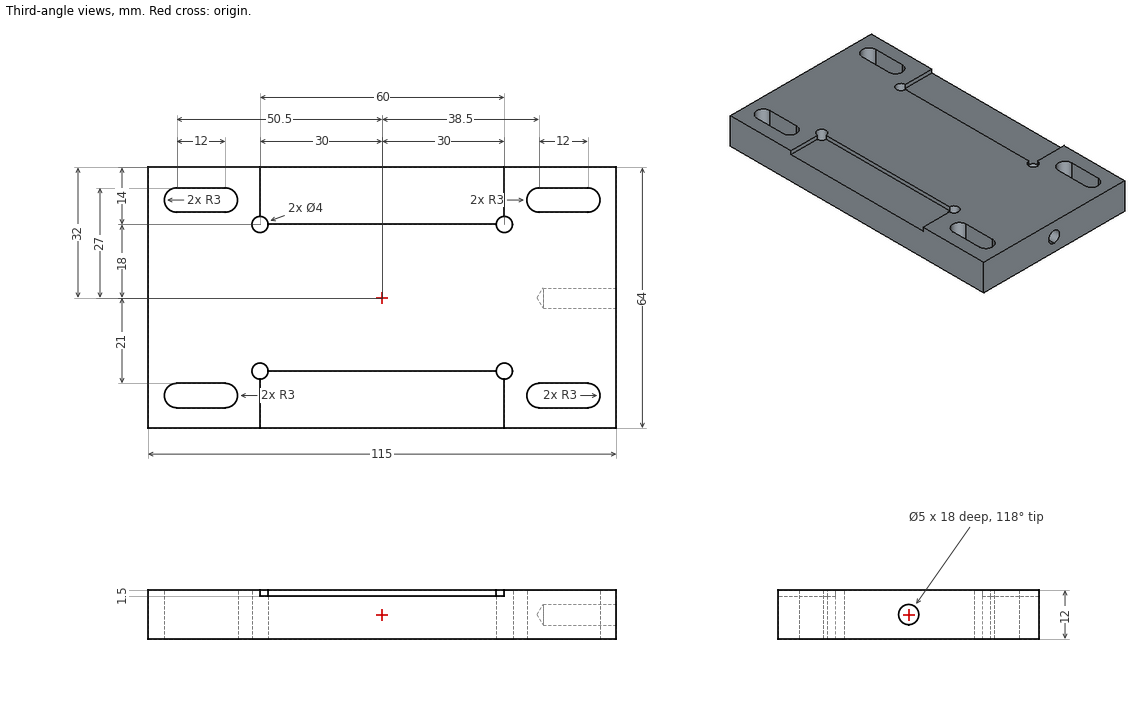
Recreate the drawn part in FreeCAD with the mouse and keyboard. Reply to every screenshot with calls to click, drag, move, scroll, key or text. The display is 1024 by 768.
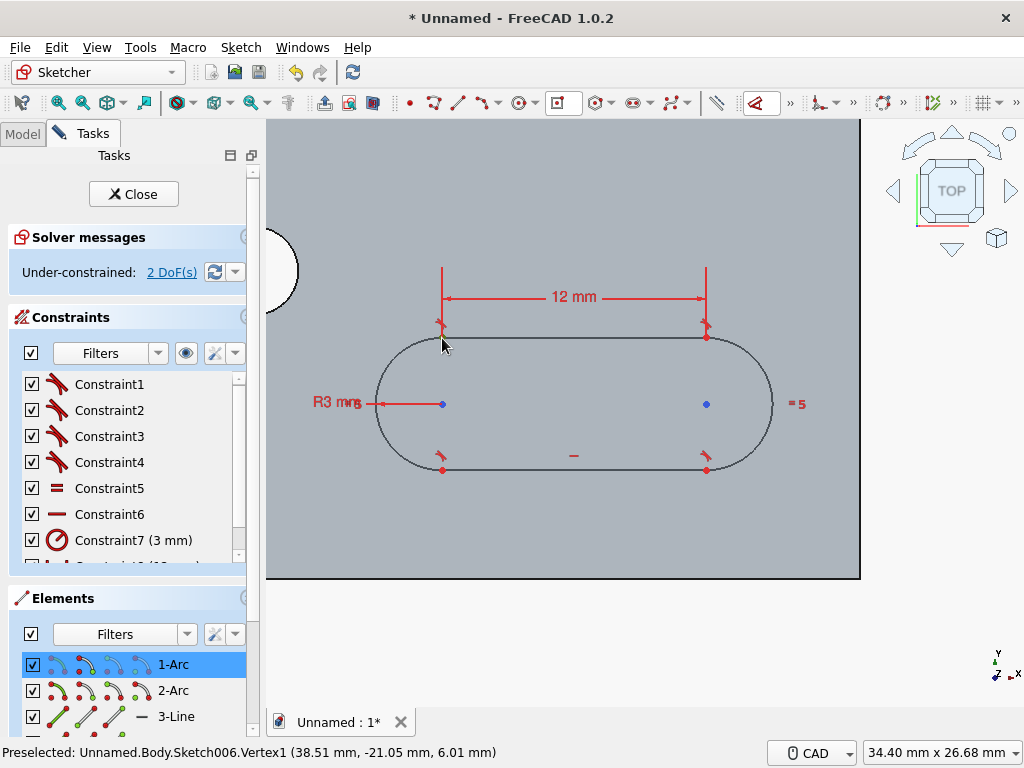
click(774, 104)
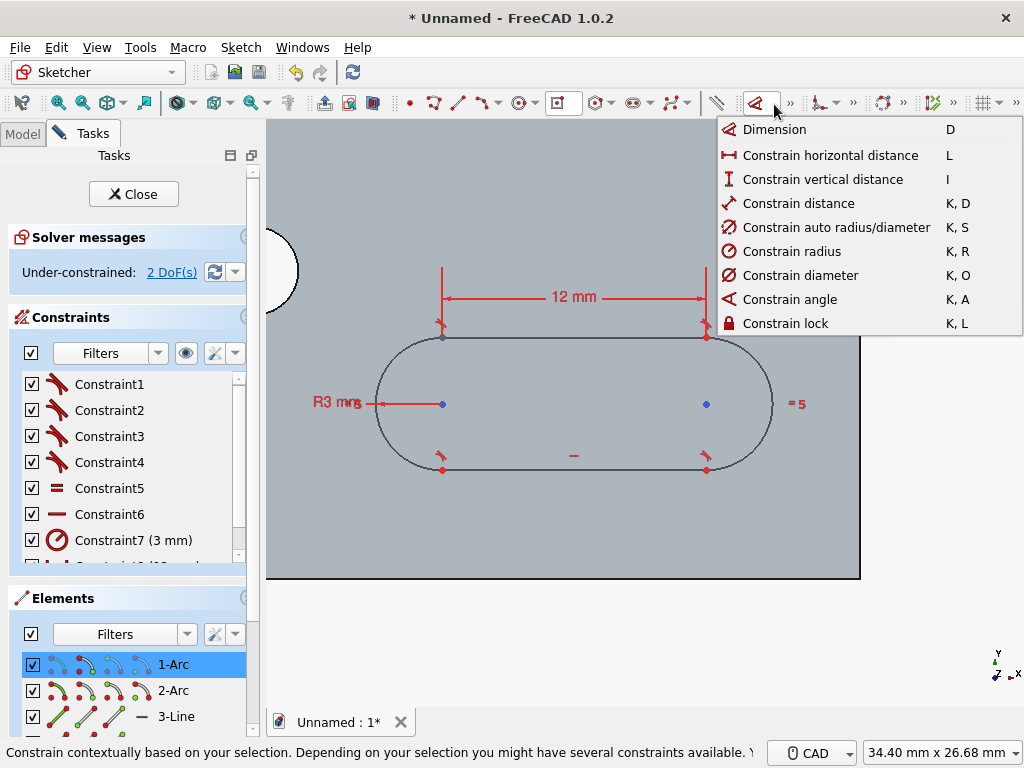
click(870, 179)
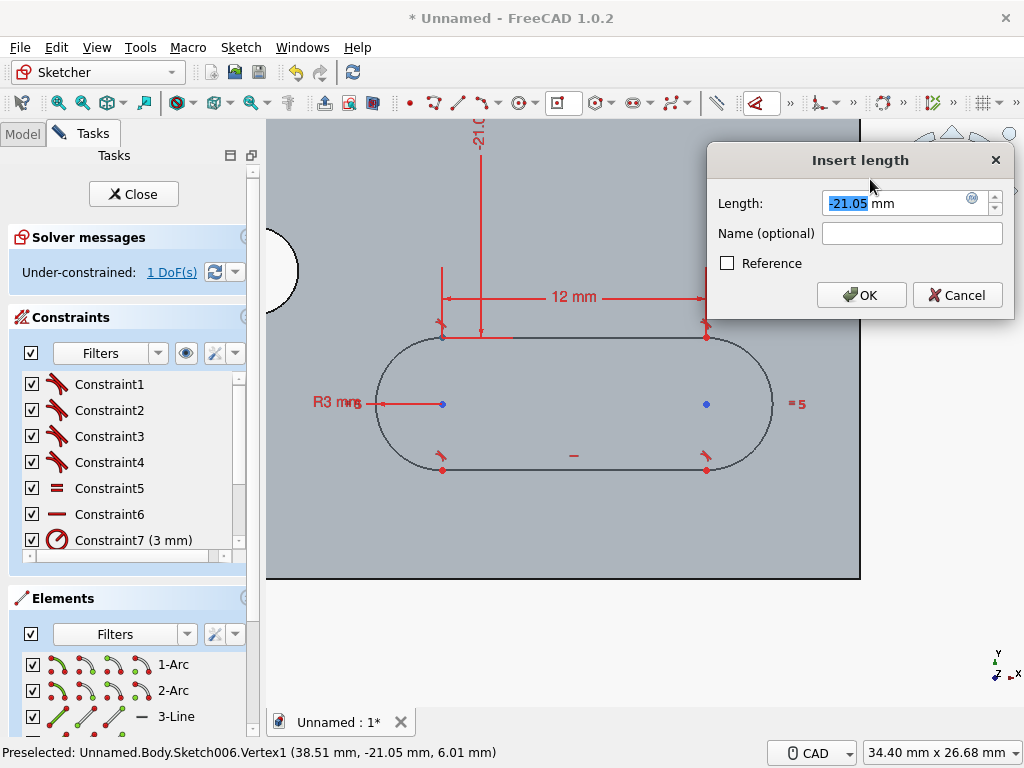
text(-21)
key(Return)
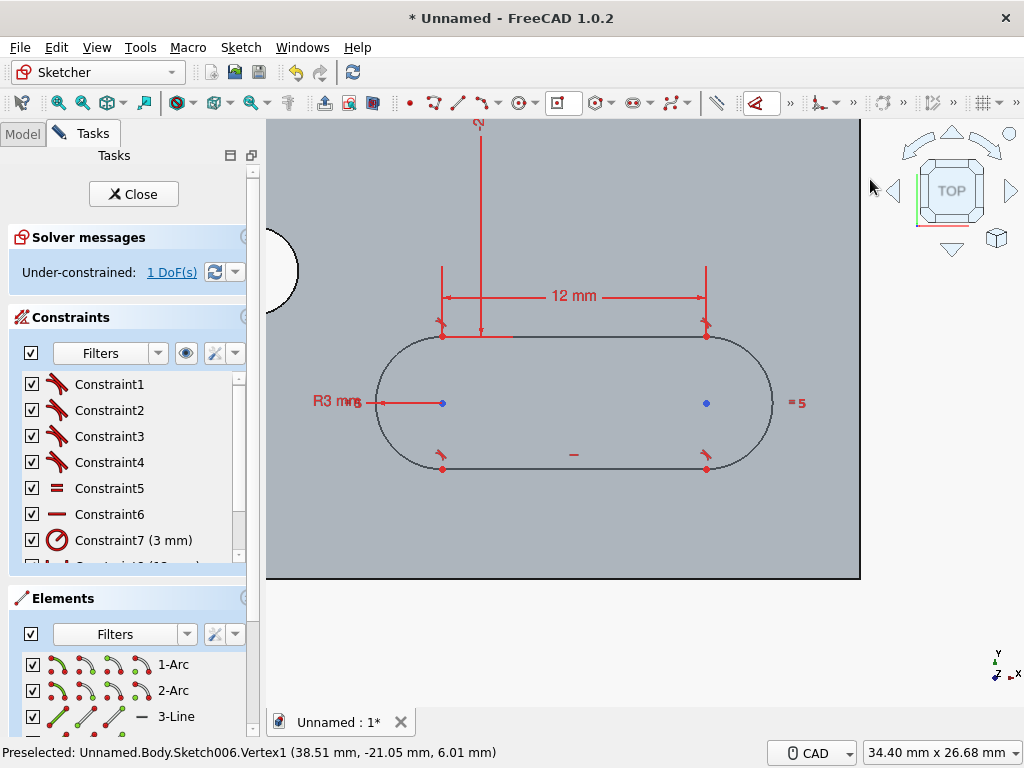
click(442, 337)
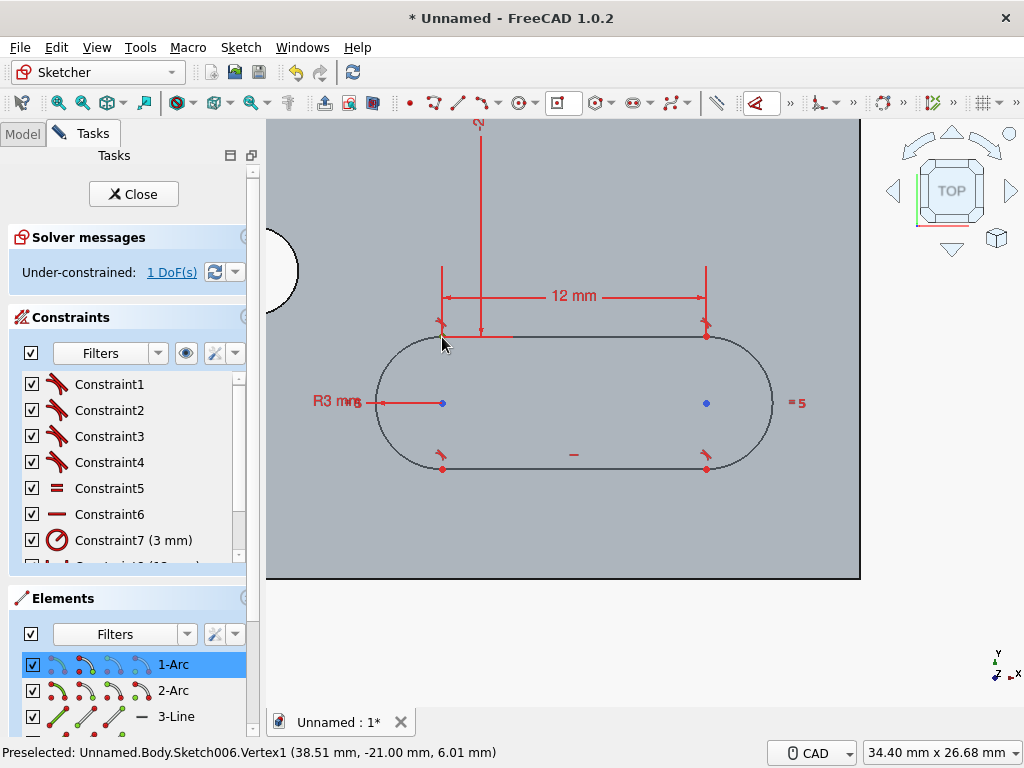
click(774, 104)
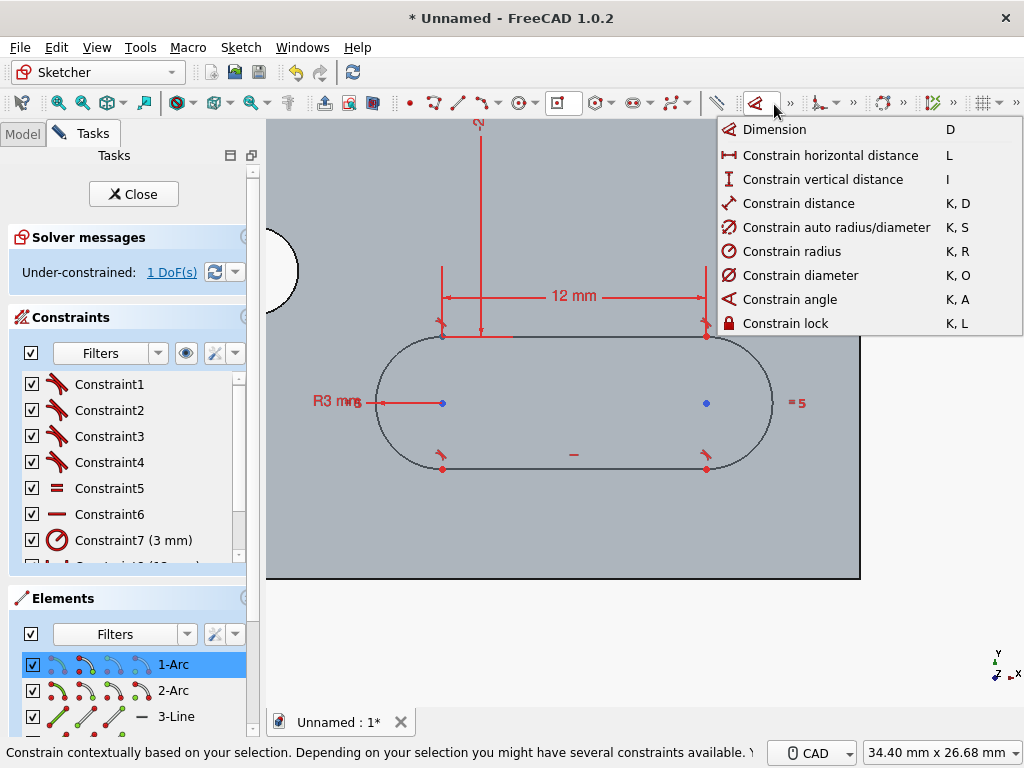
click(870, 155)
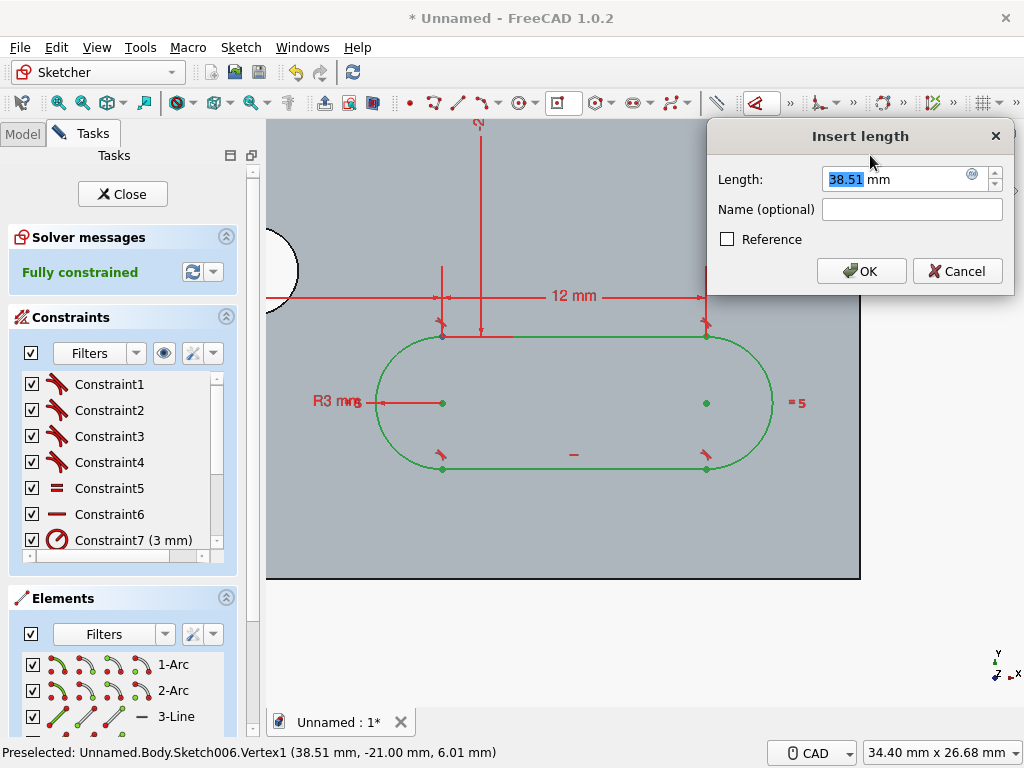
text(38.5)
key(Return)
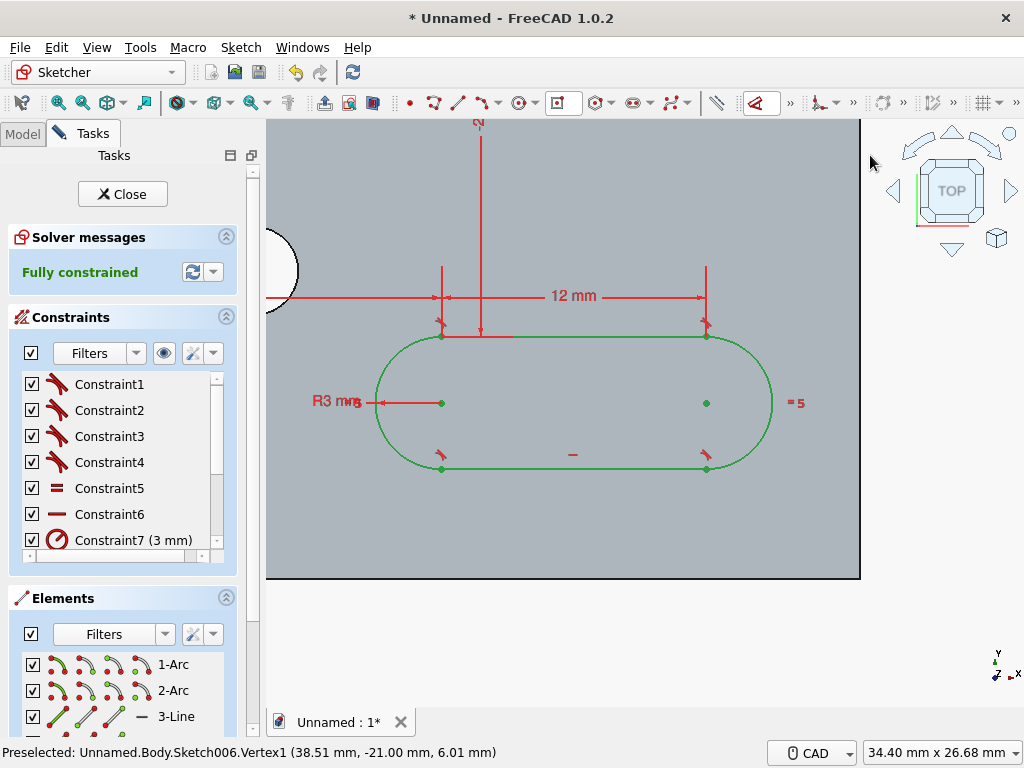
click(123, 194)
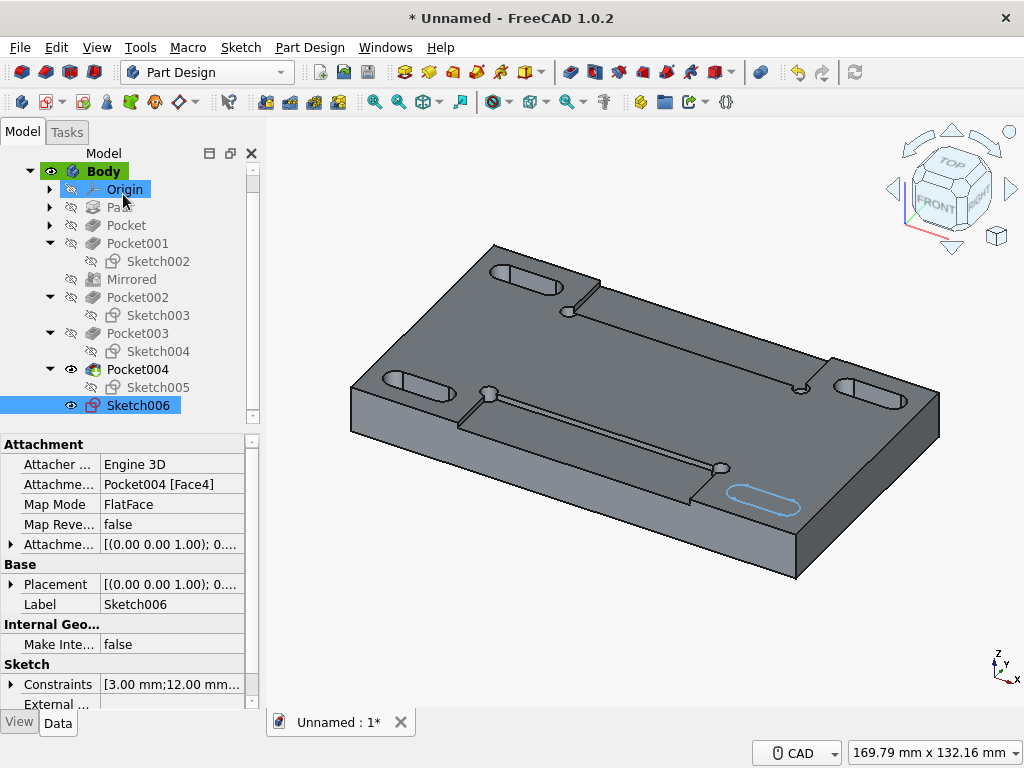
click(572, 72)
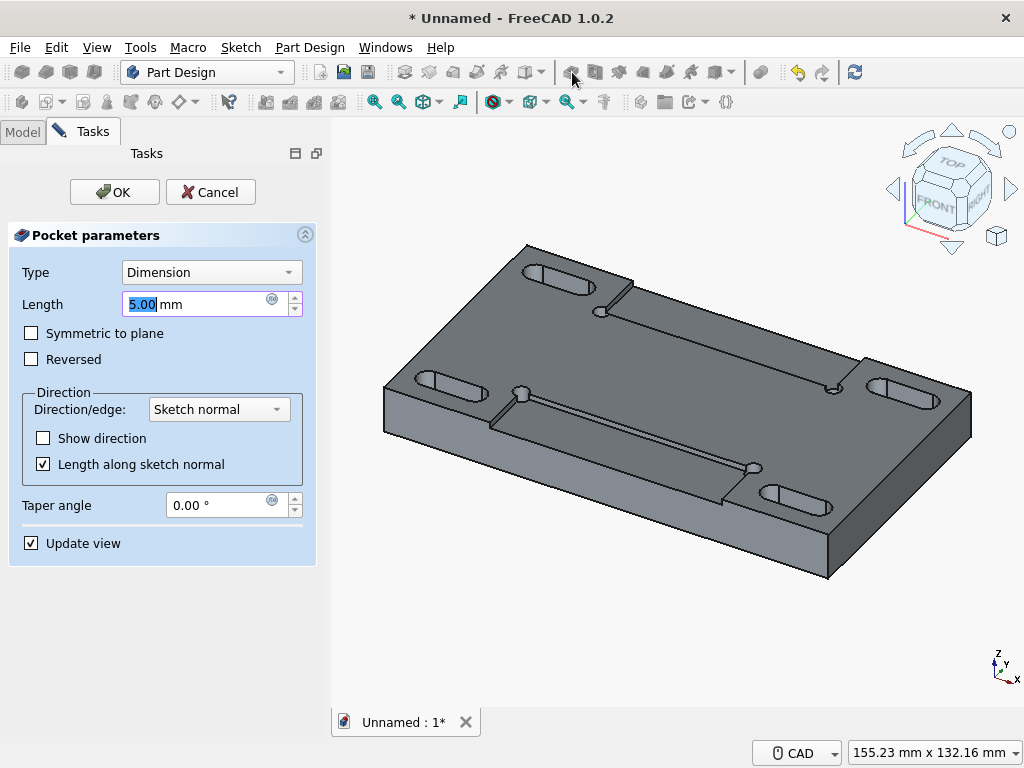
click(212, 272)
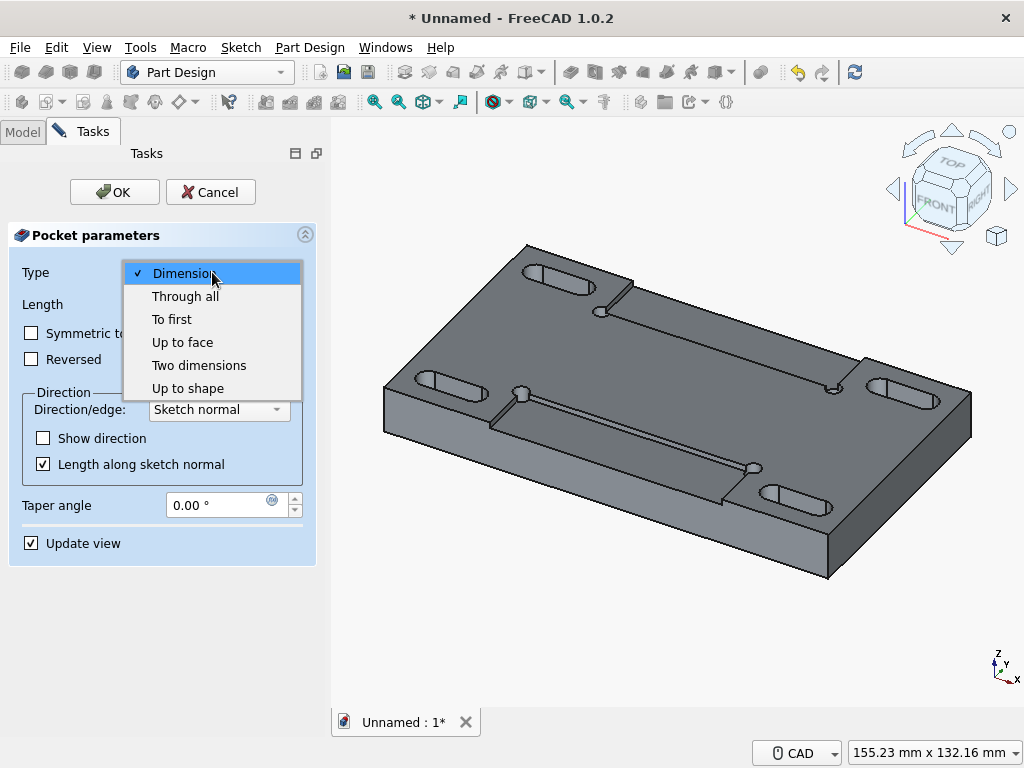
click(212, 320)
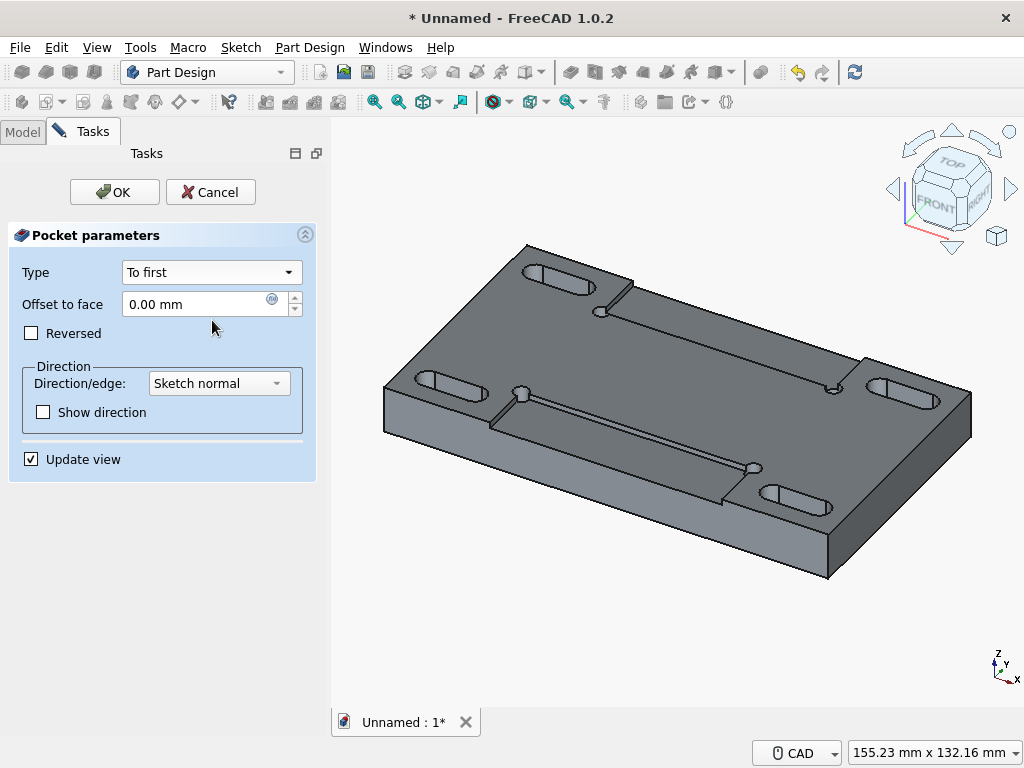
click(115, 192)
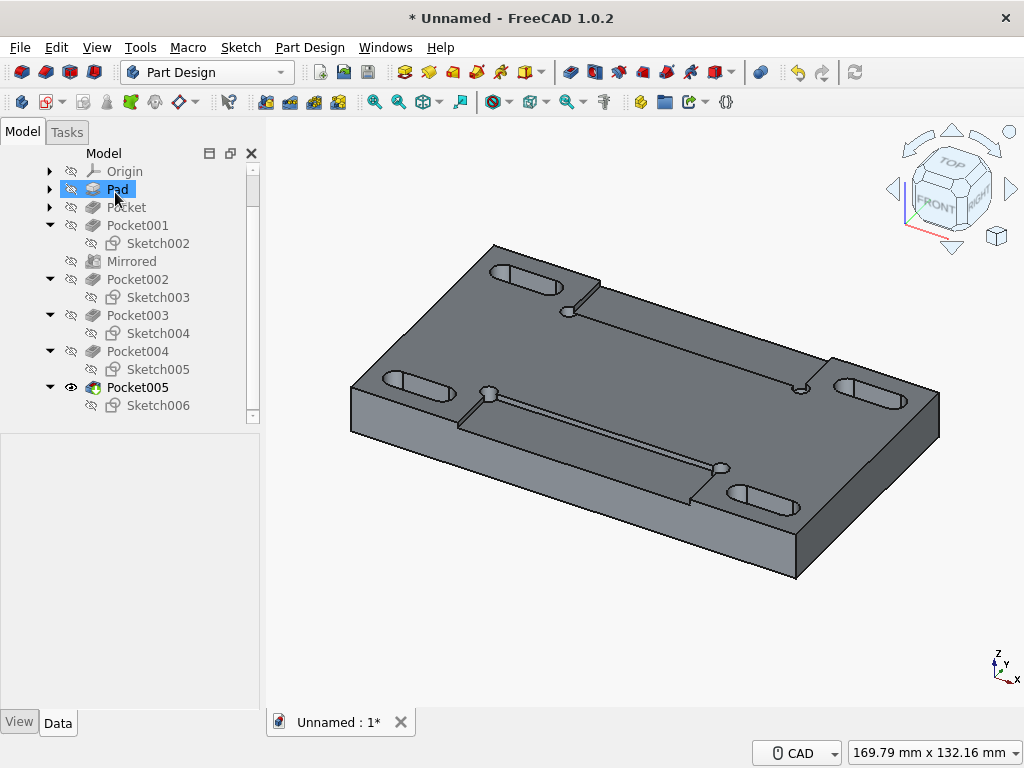
click(908, 444)